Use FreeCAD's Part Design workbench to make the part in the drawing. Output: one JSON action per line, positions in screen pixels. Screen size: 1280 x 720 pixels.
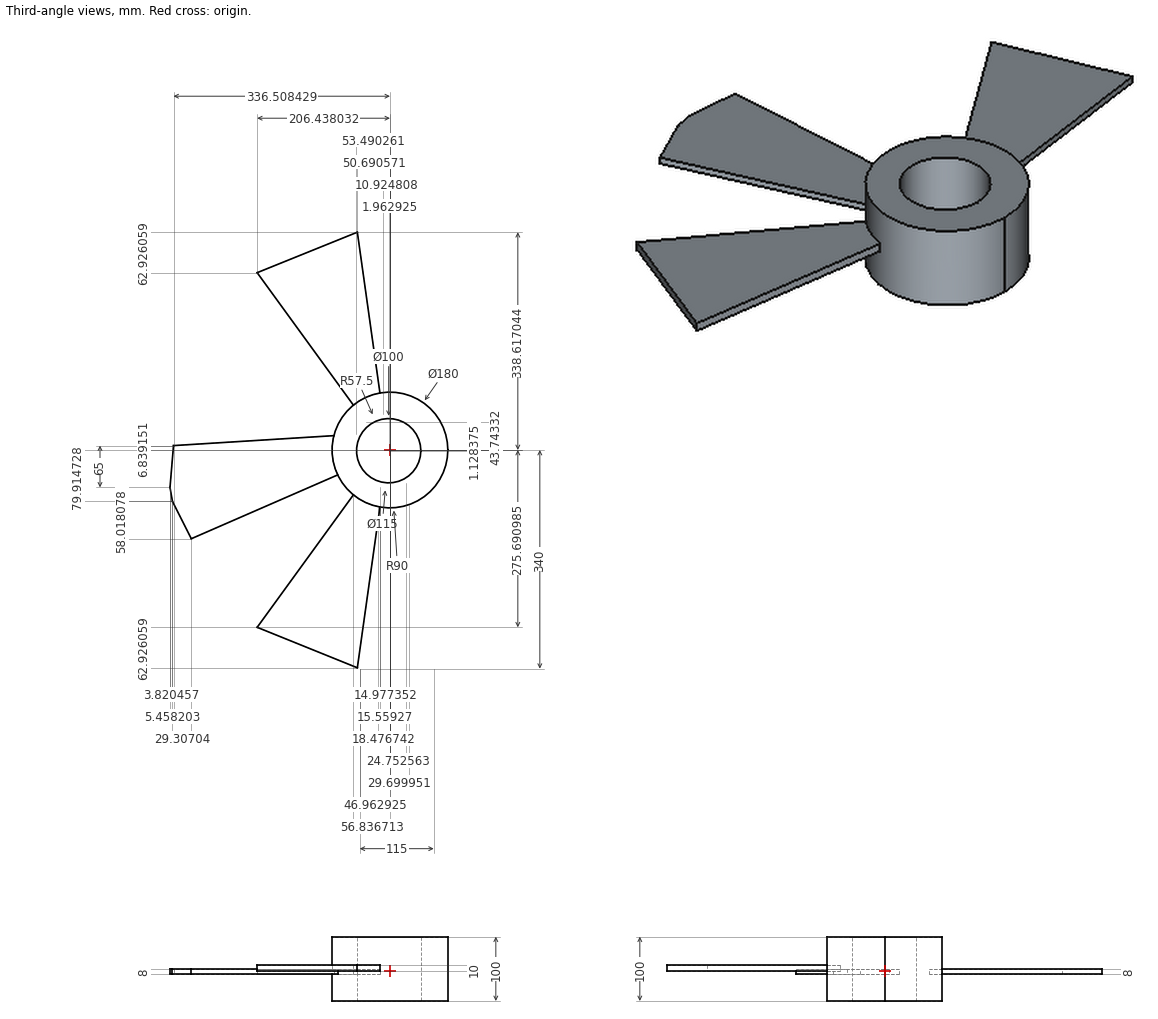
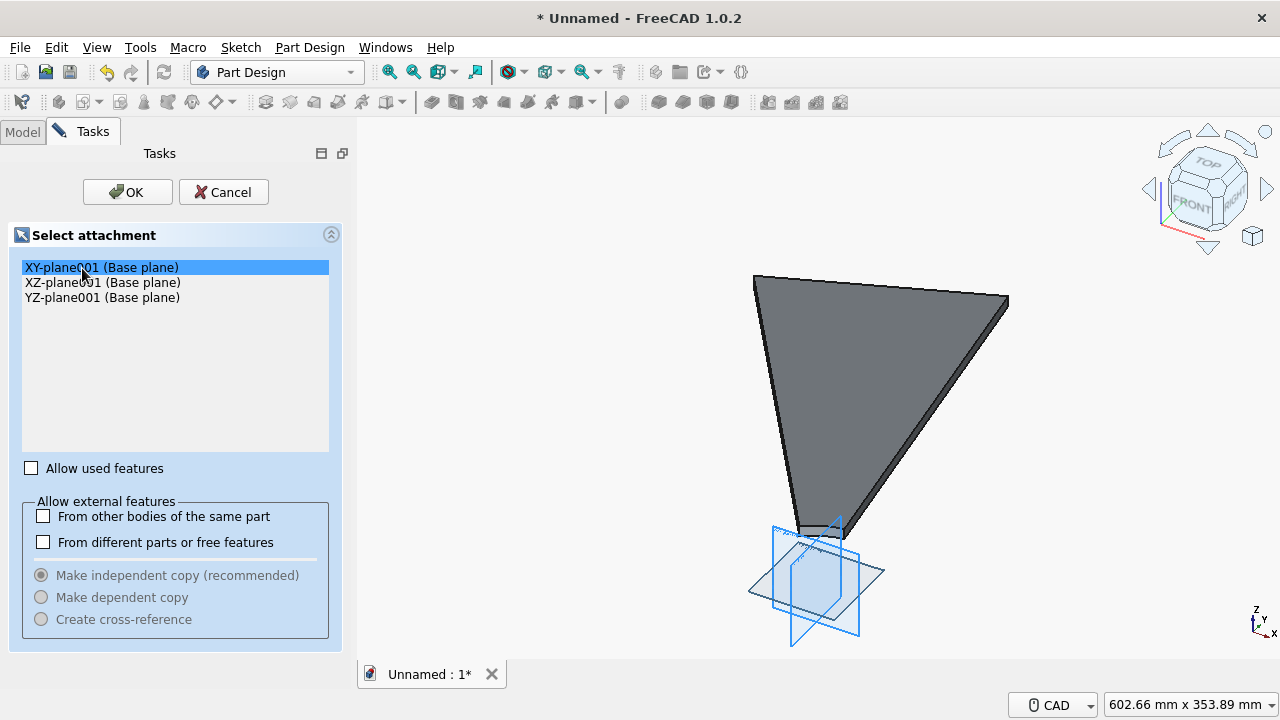
{"action": "left_click", "coordinate": [128, 192]}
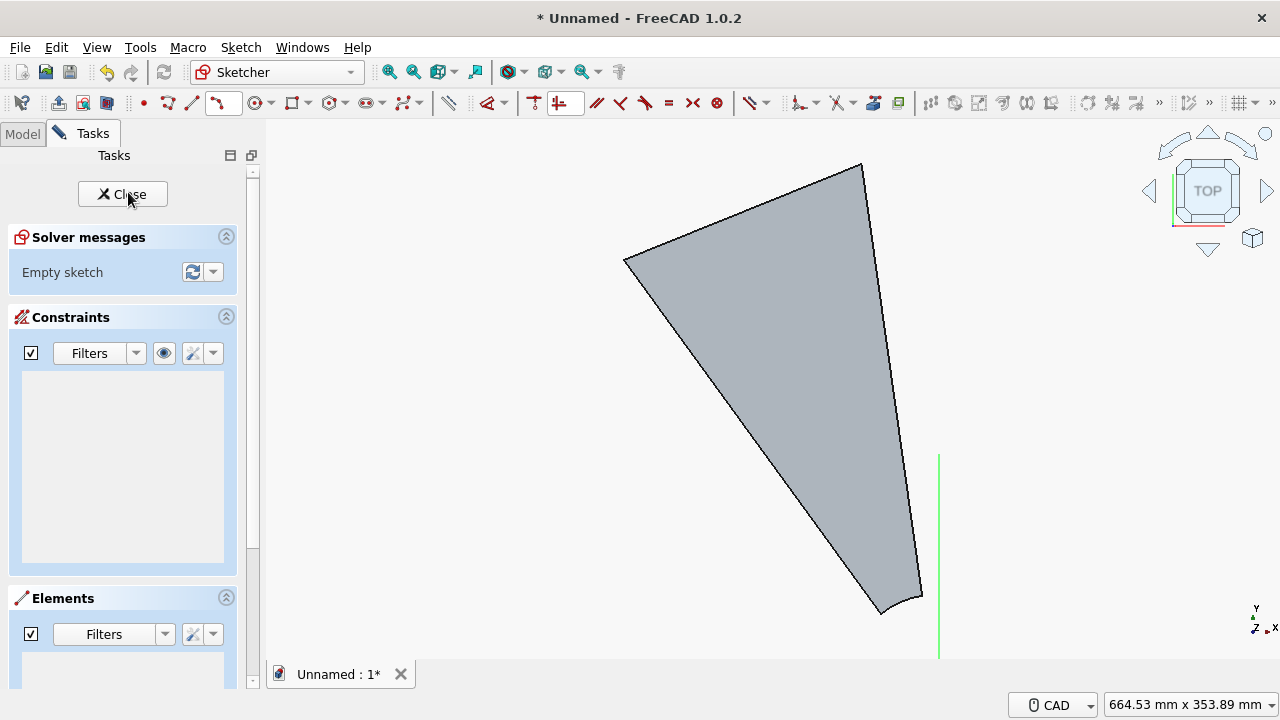
{"action": "scroll", "coordinate": [704, 389], "scroll_direction": "down", "scroll_amount": 5}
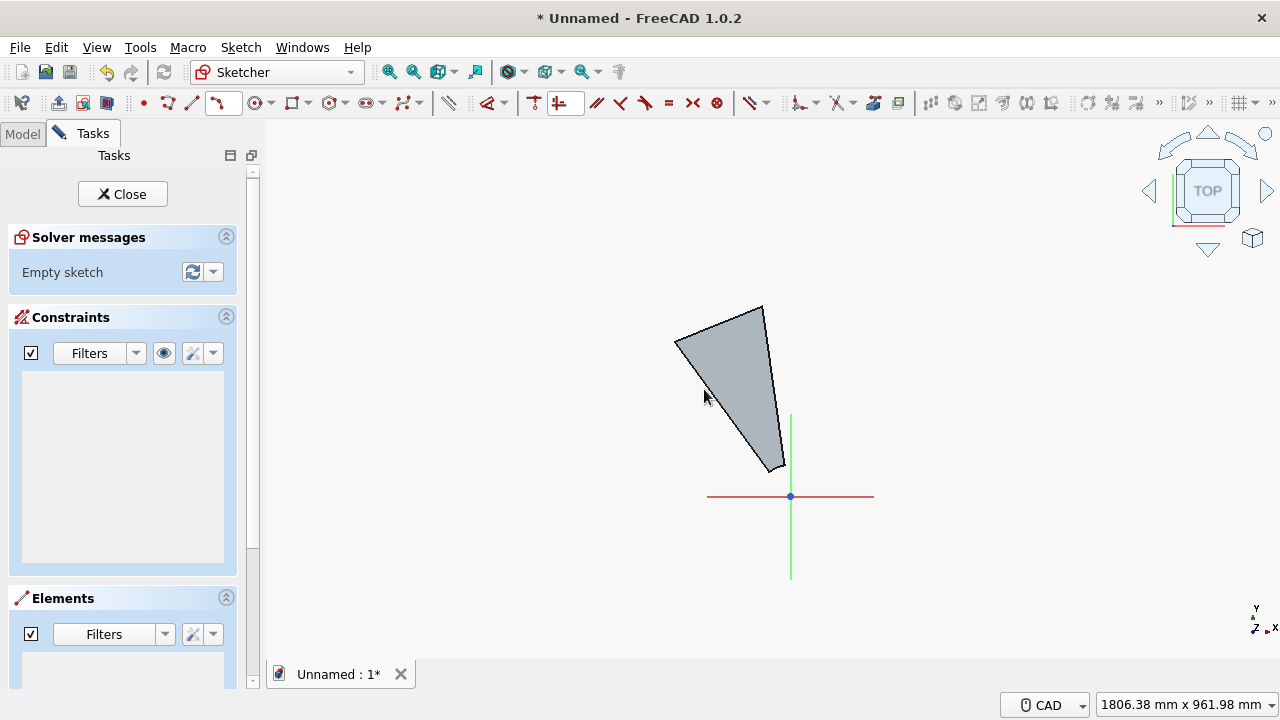
{"action": "scroll", "coordinate": [690, 589], "scroll_direction": "up", "scroll_amount": 6}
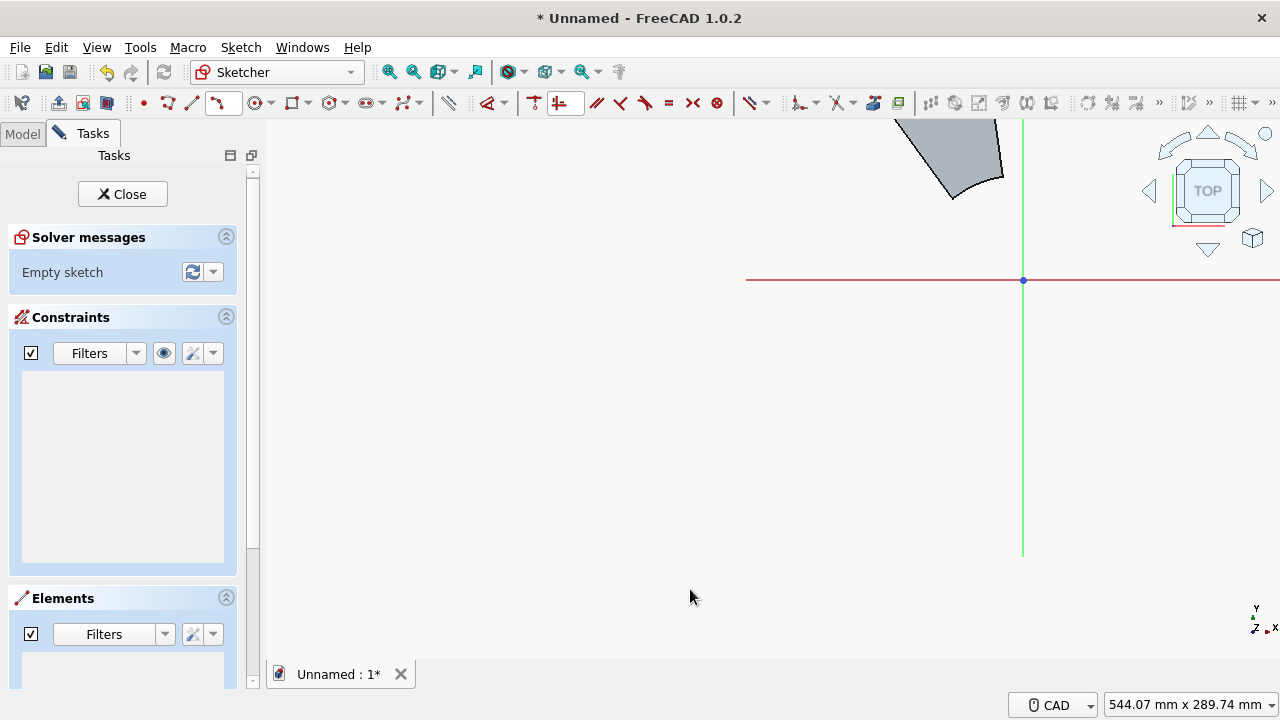
{"action": "left_click", "coordinate": [168, 104]}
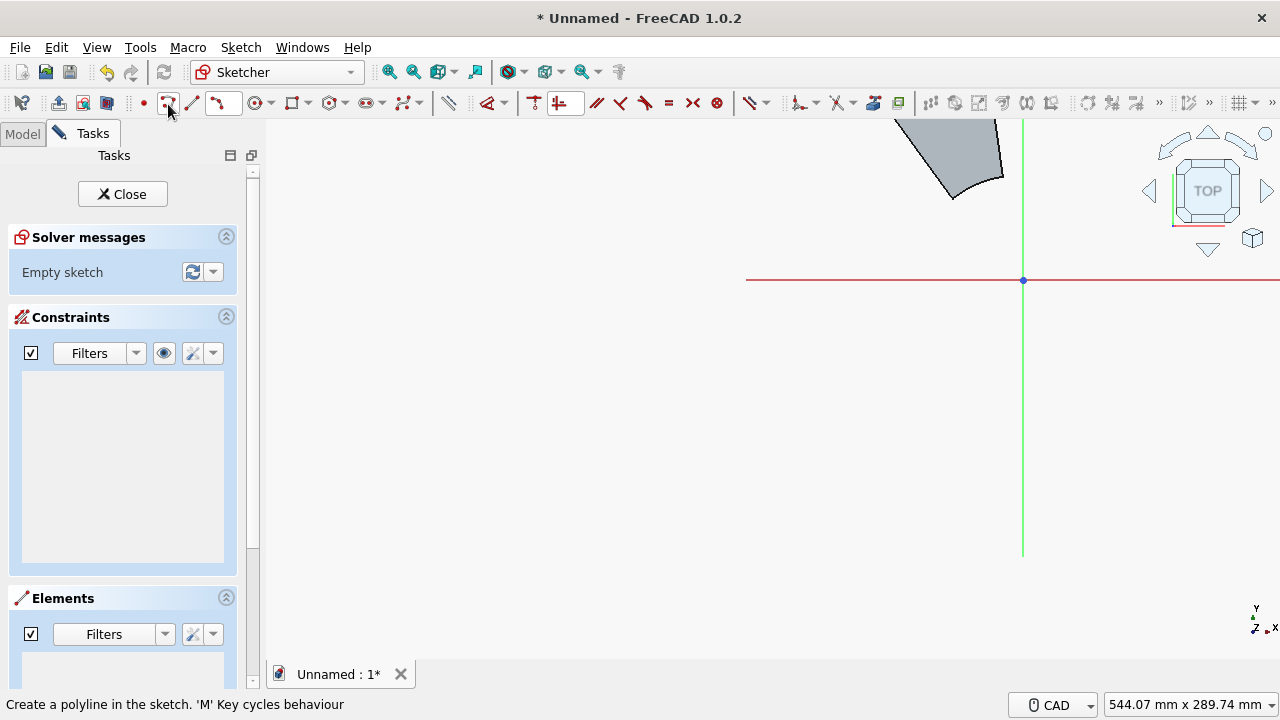
{"action": "left_click", "coordinate": [924, 235]}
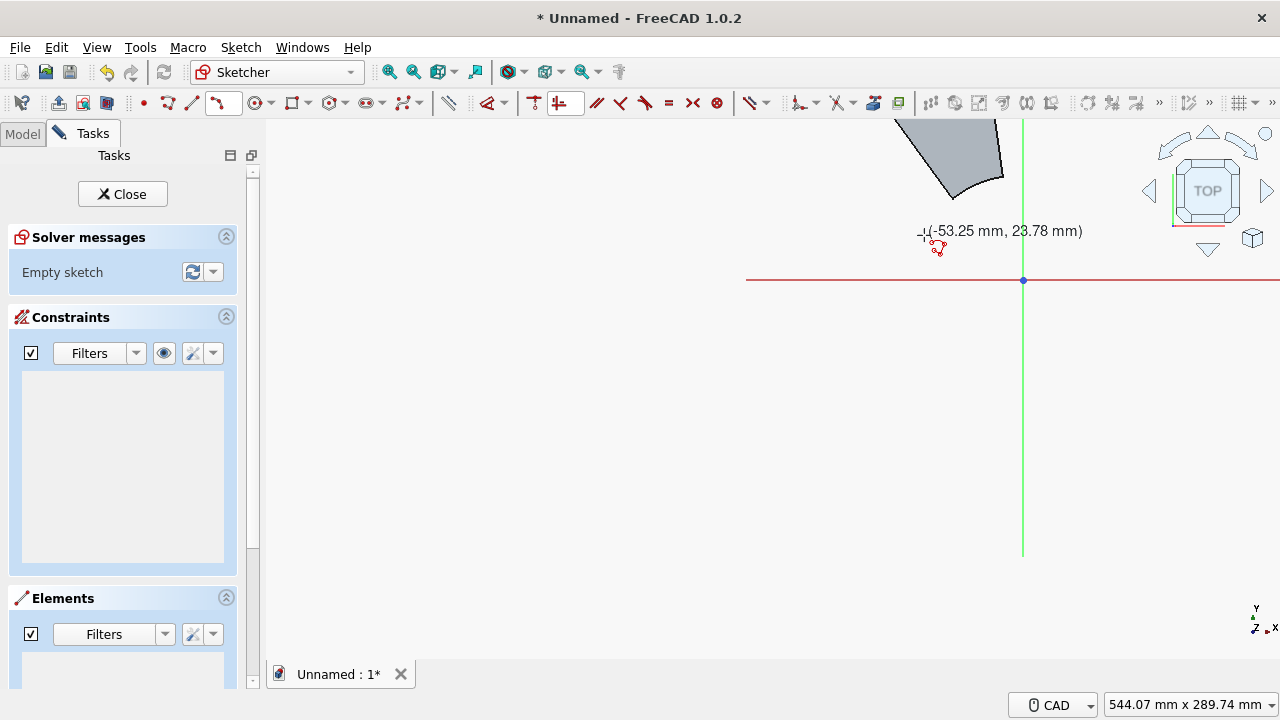
{"action": "scroll", "coordinate": [396, 268], "scroll_direction": "up", "scroll_amount": 2}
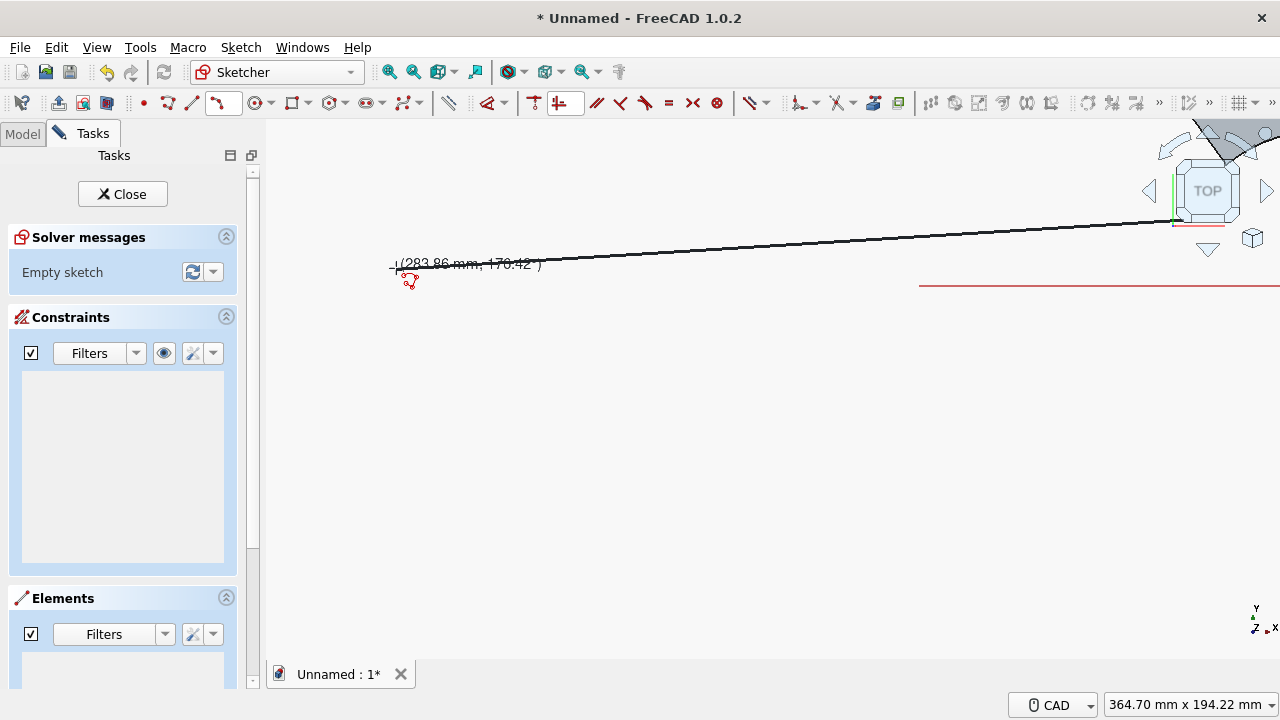
{"action": "left_click", "coordinate": [396, 267]}
{"action": "left_click", "coordinate": [381, 448]}
{"action": "left_click", "coordinate": [392, 508]}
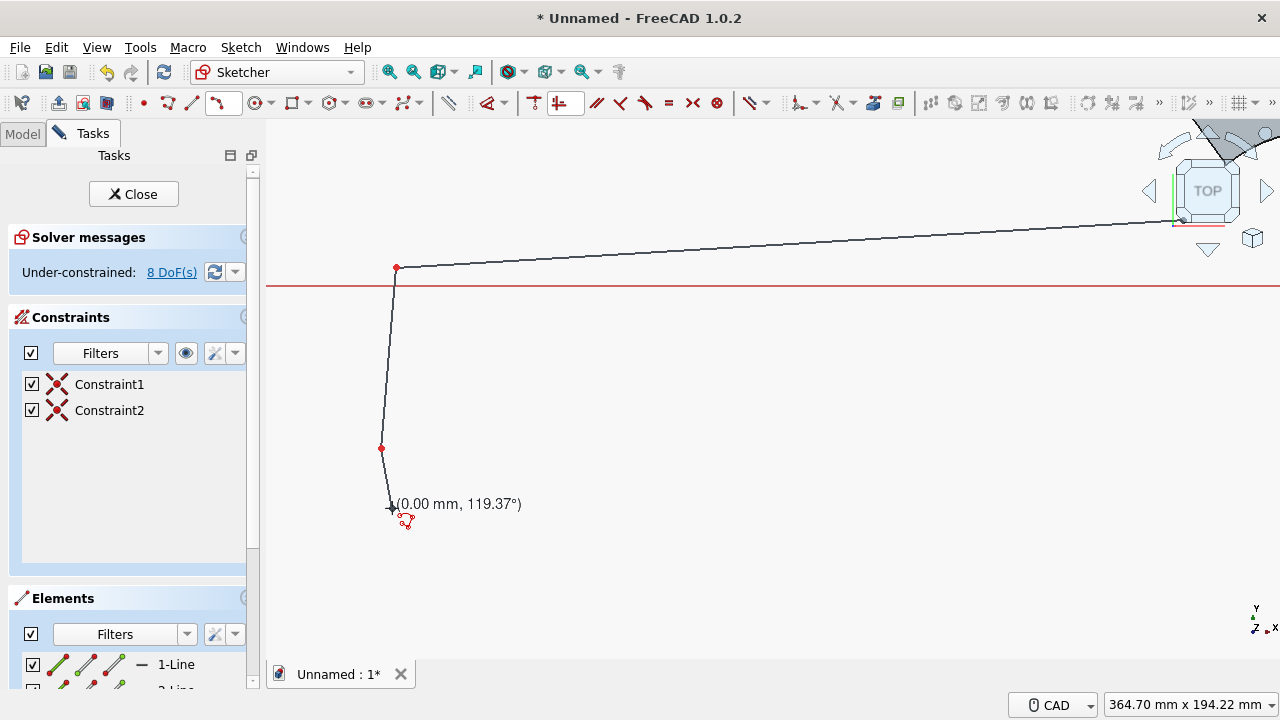
{"action": "scroll", "coordinate": [396, 277], "scroll_direction": "down", "scroll_amount": 2}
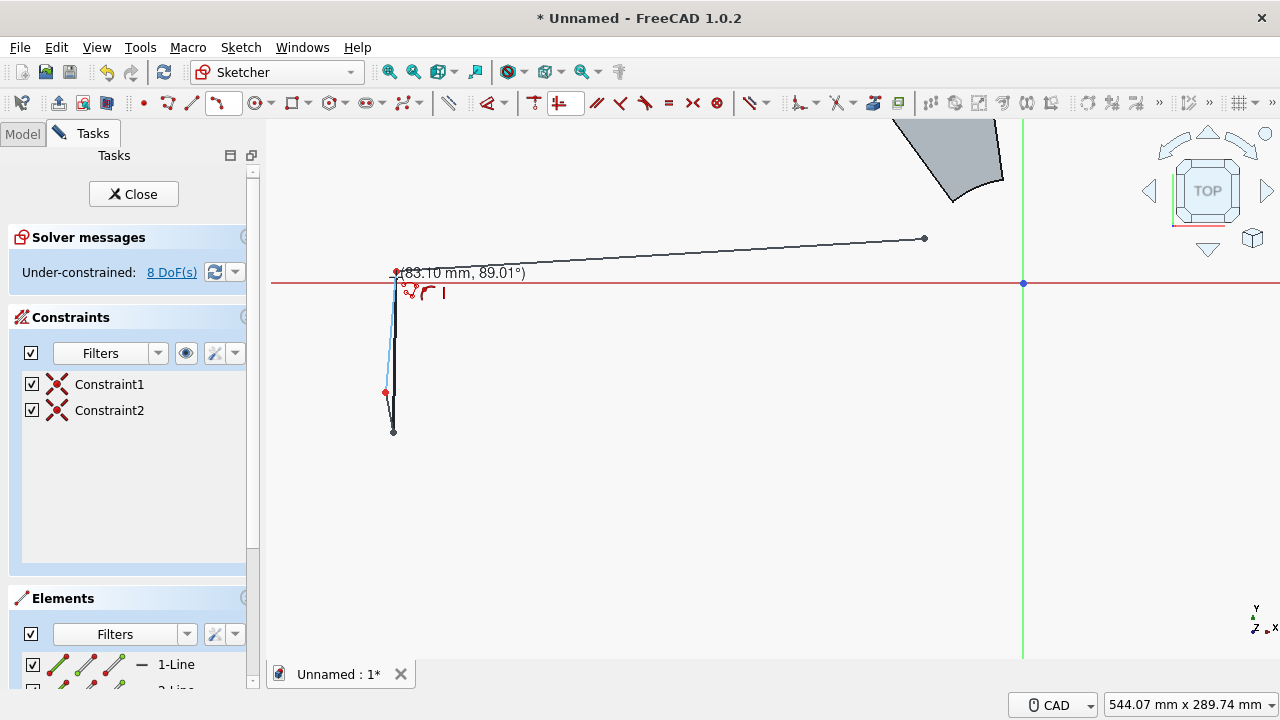
{"action": "left_click", "coordinate": [448, 540]}
{"action": "left_click", "coordinate": [924, 333]}
{"action": "right_click", "coordinate": [924, 333]}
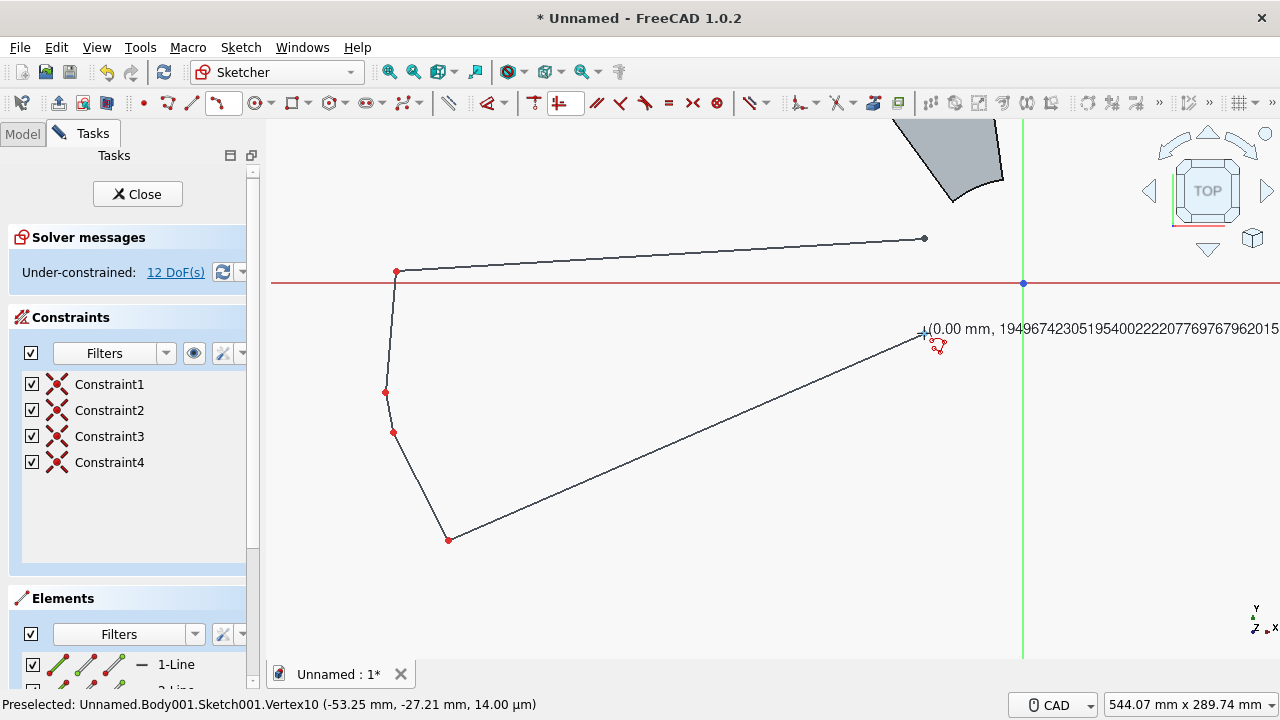
{"action": "left_click", "coordinate": [218, 104]}